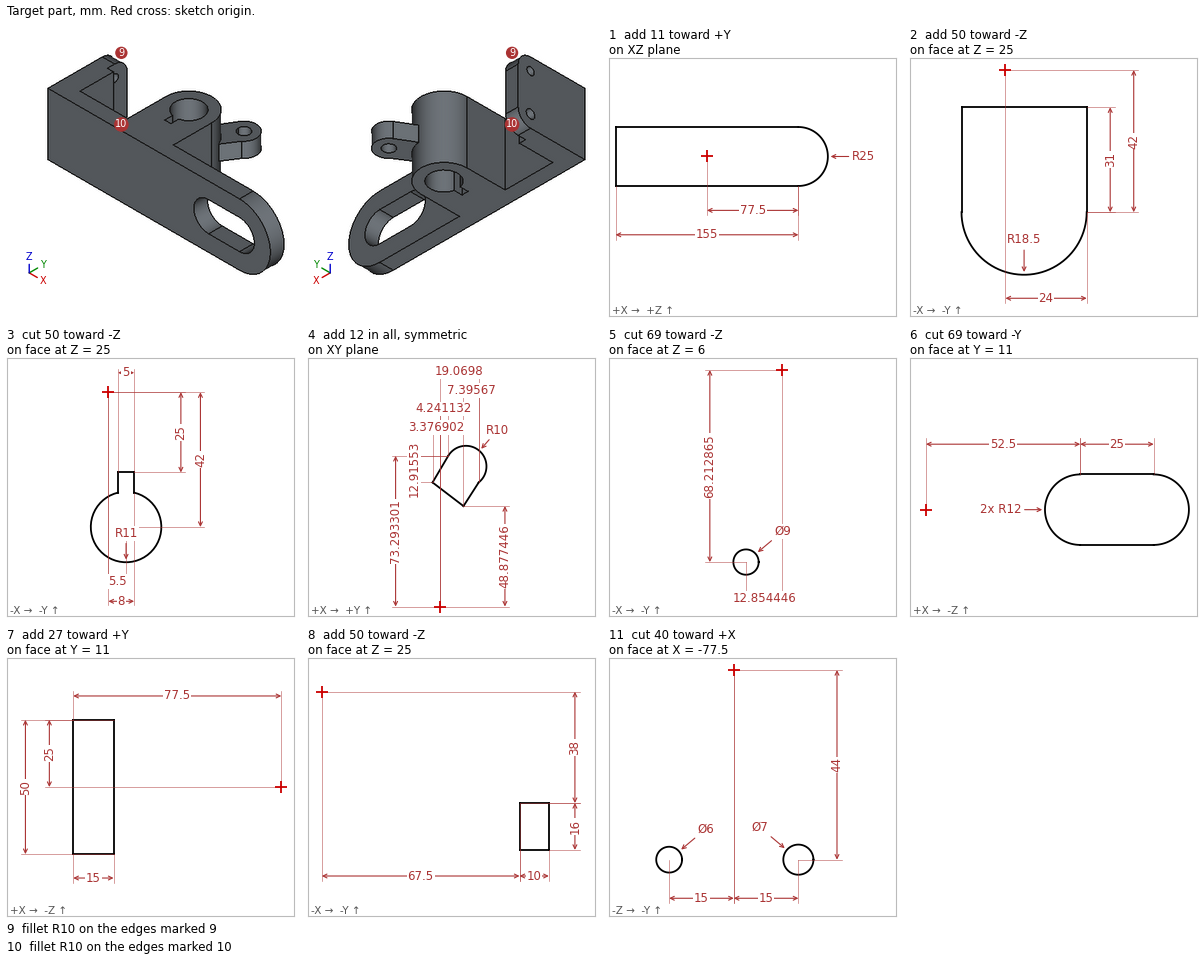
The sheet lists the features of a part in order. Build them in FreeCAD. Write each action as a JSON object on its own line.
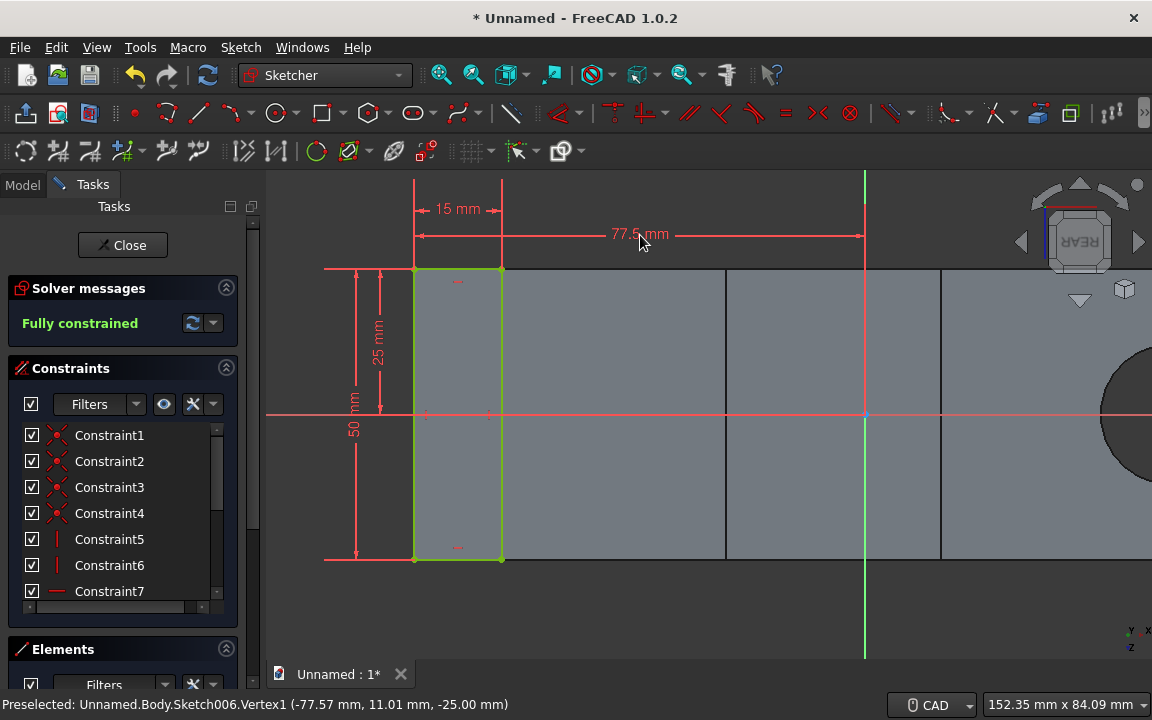
{"action": "left_click", "coordinate": [123, 245]}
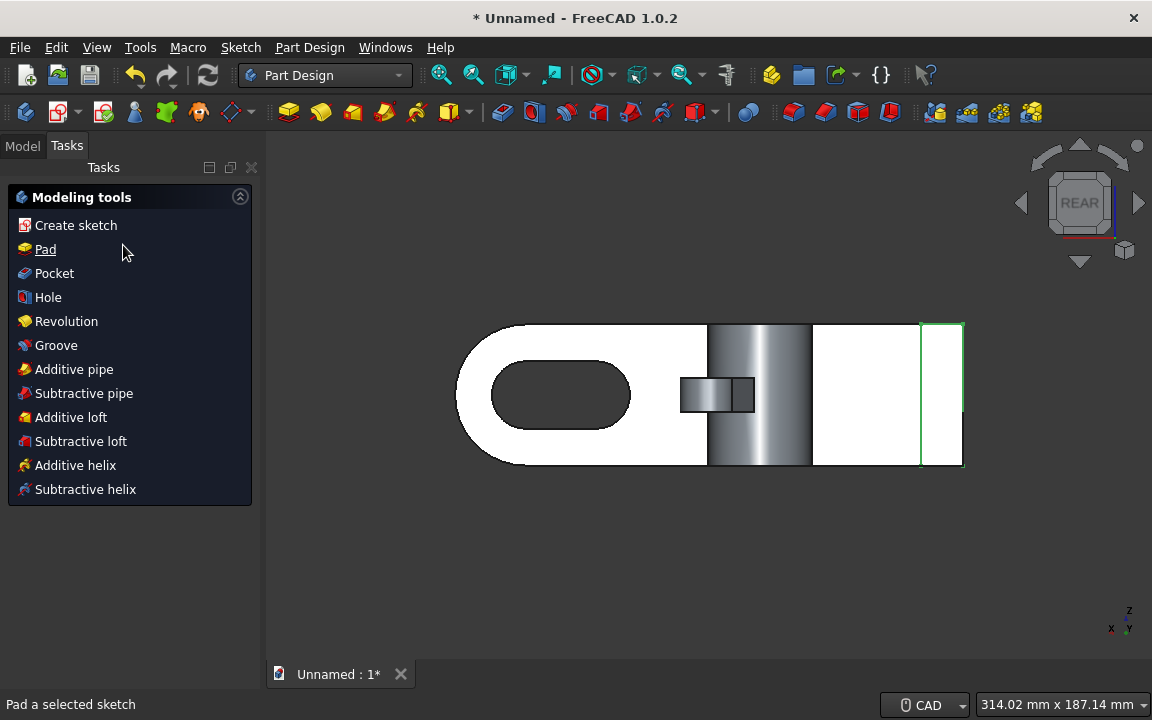
{"action": "left_click", "coordinate": [290, 112]}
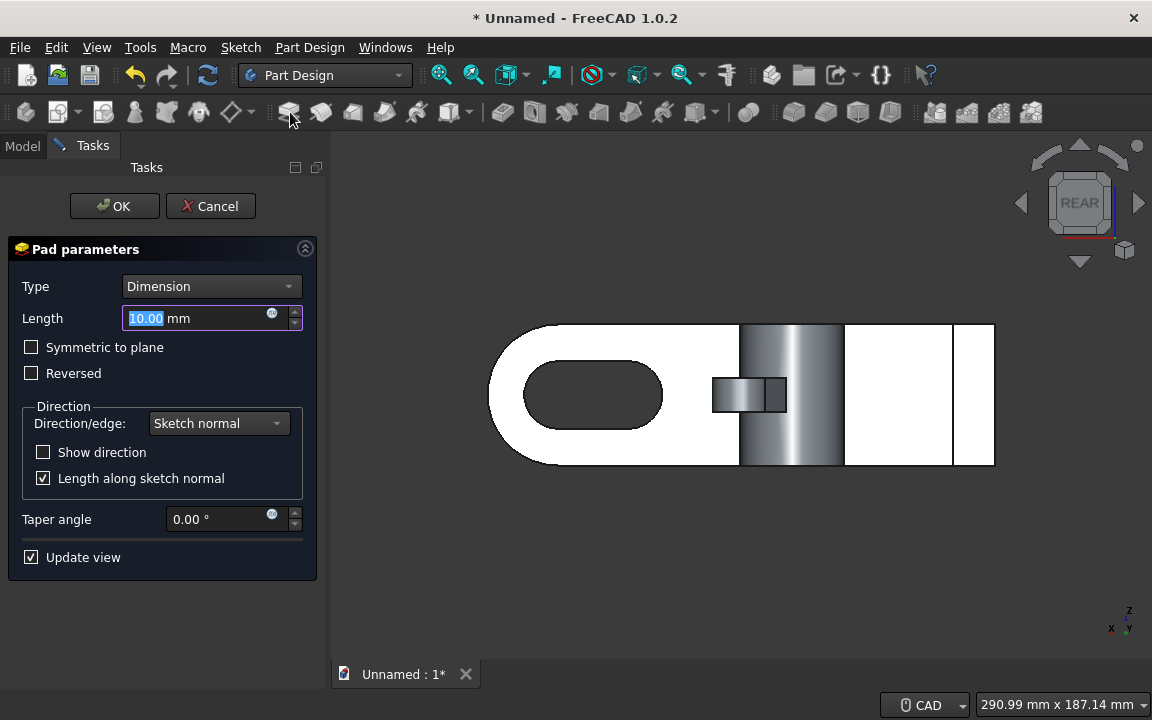
{"action": "type", "text": "27"}
{"action": "key", "text": "Tab"}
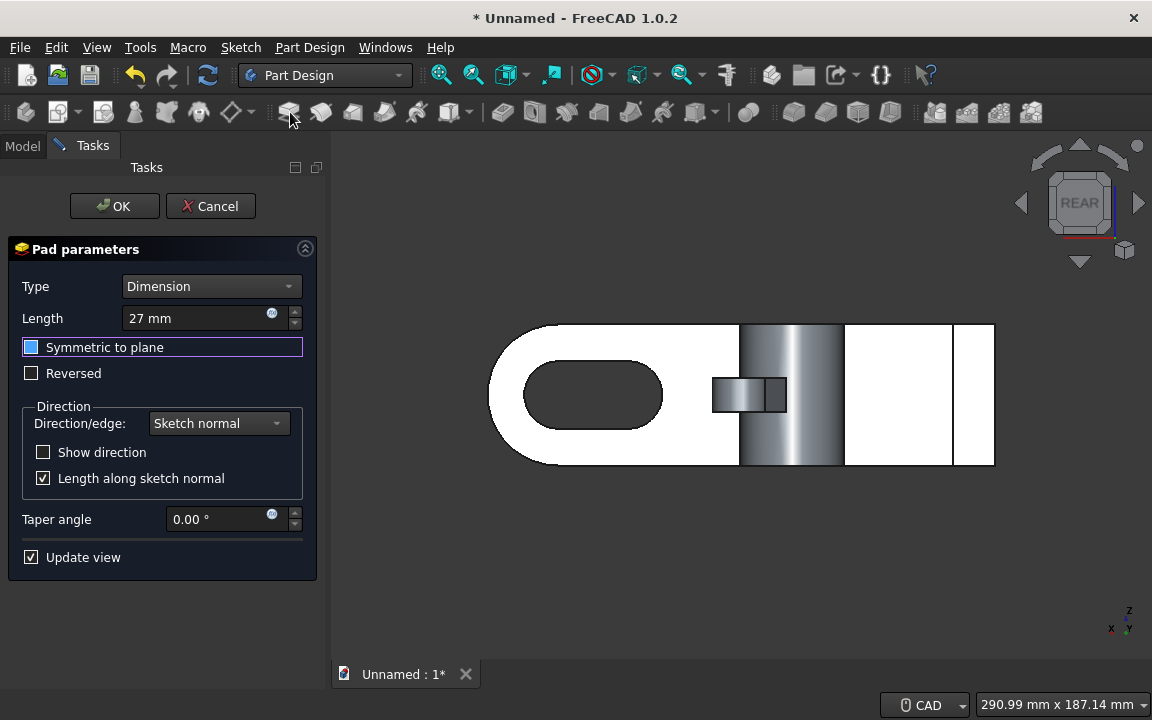
{"action": "left_click", "coordinate": [115, 206]}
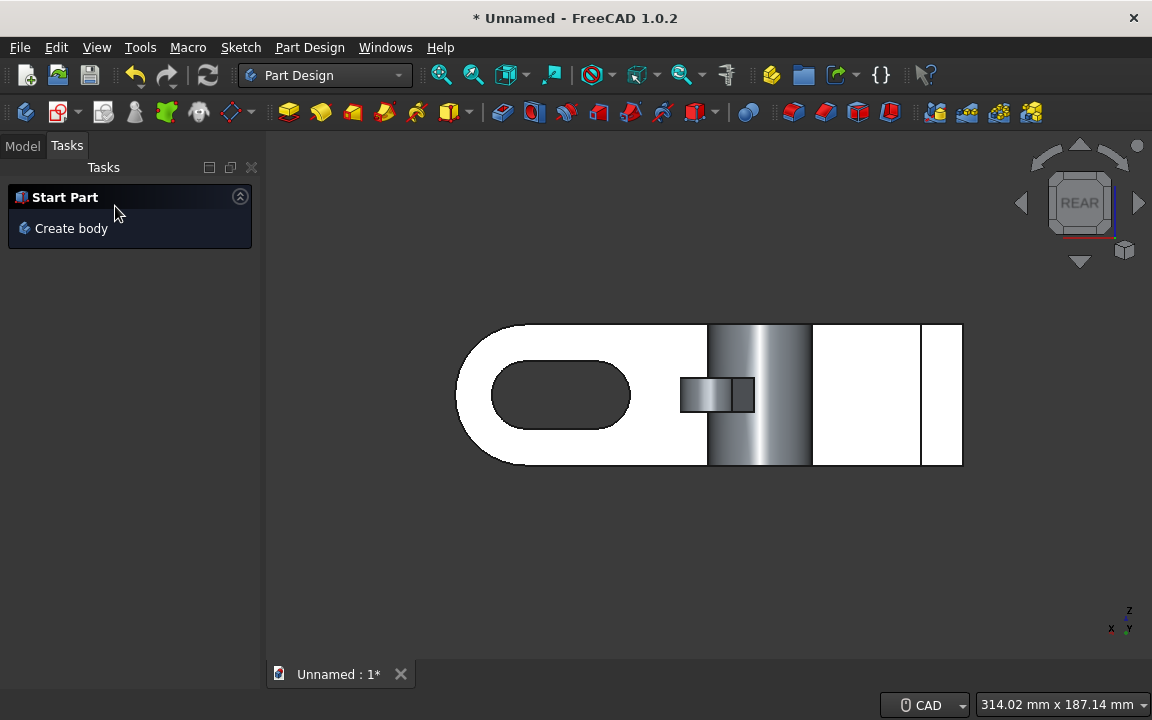
{"action": "key", "text": "0"}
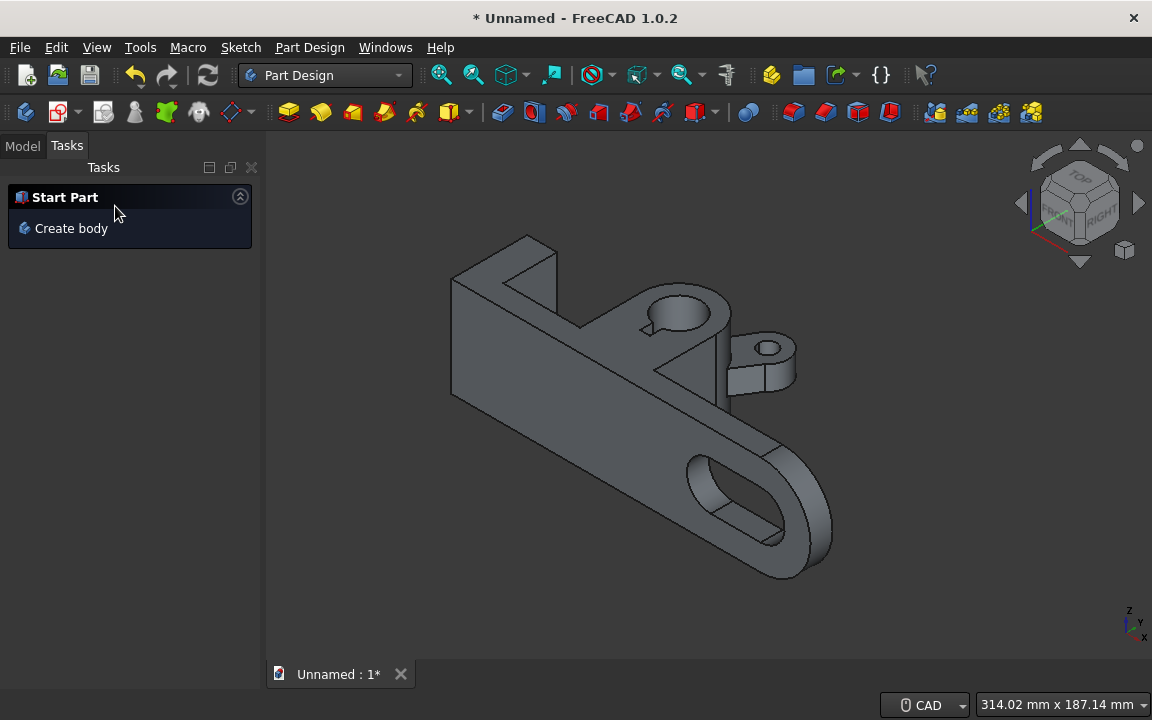
{"action": "left_click", "coordinate": [632, 352]}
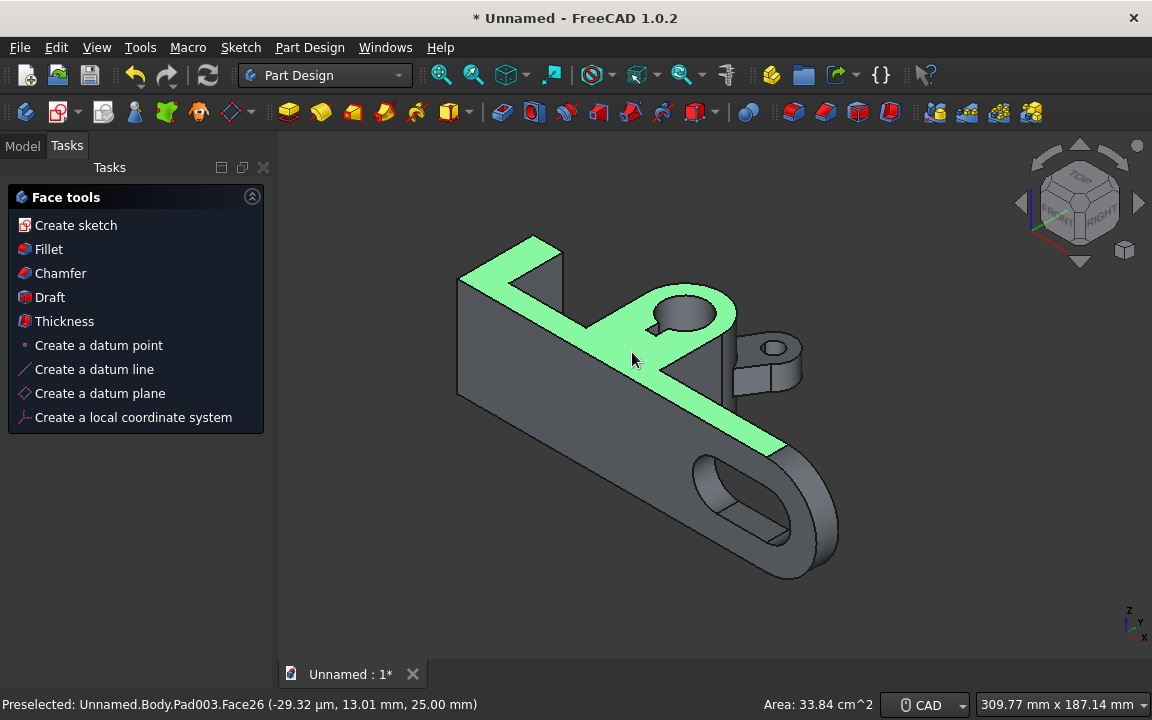
{"action": "left_click", "coordinate": [58, 112]}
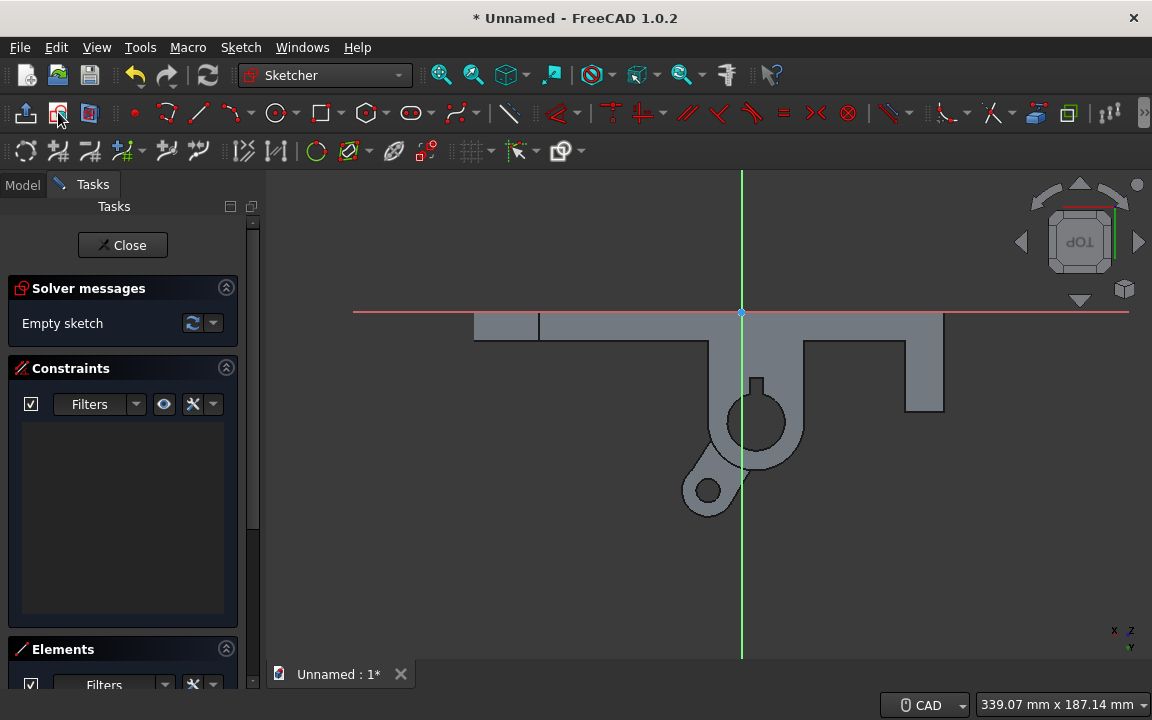
{"action": "scroll", "coordinate": [977, 435], "scroll_direction": "up", "scroll_amount": 10}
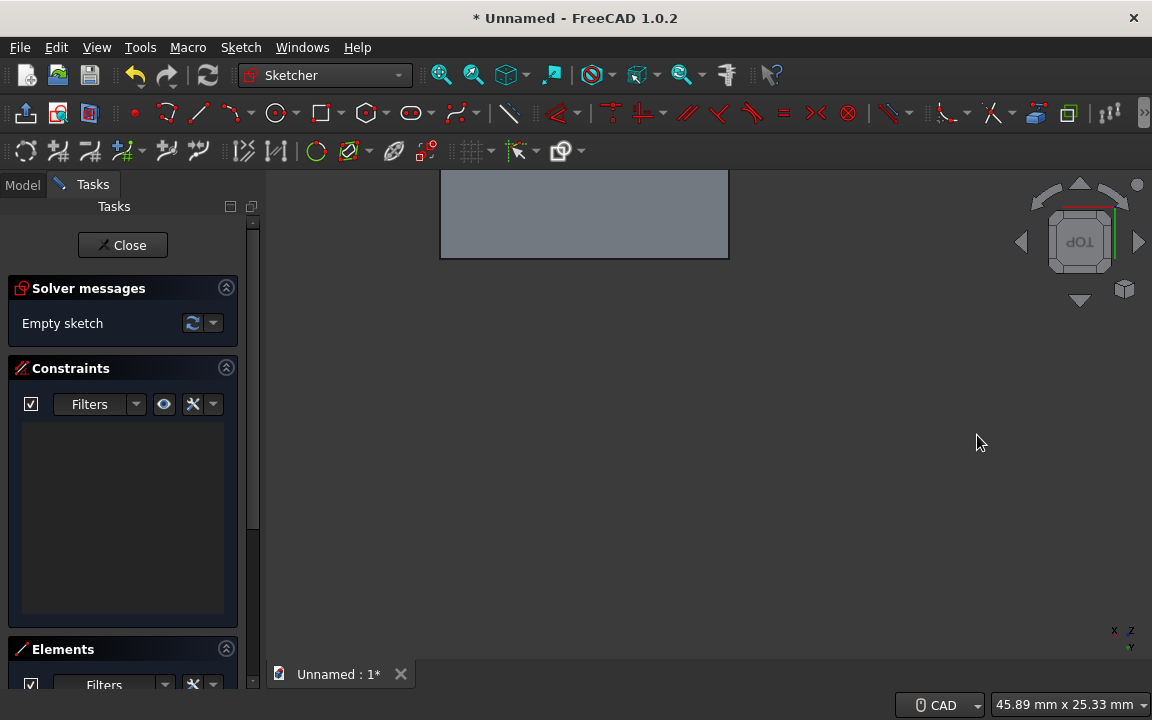
{"action": "left_click", "coordinate": [322, 114]}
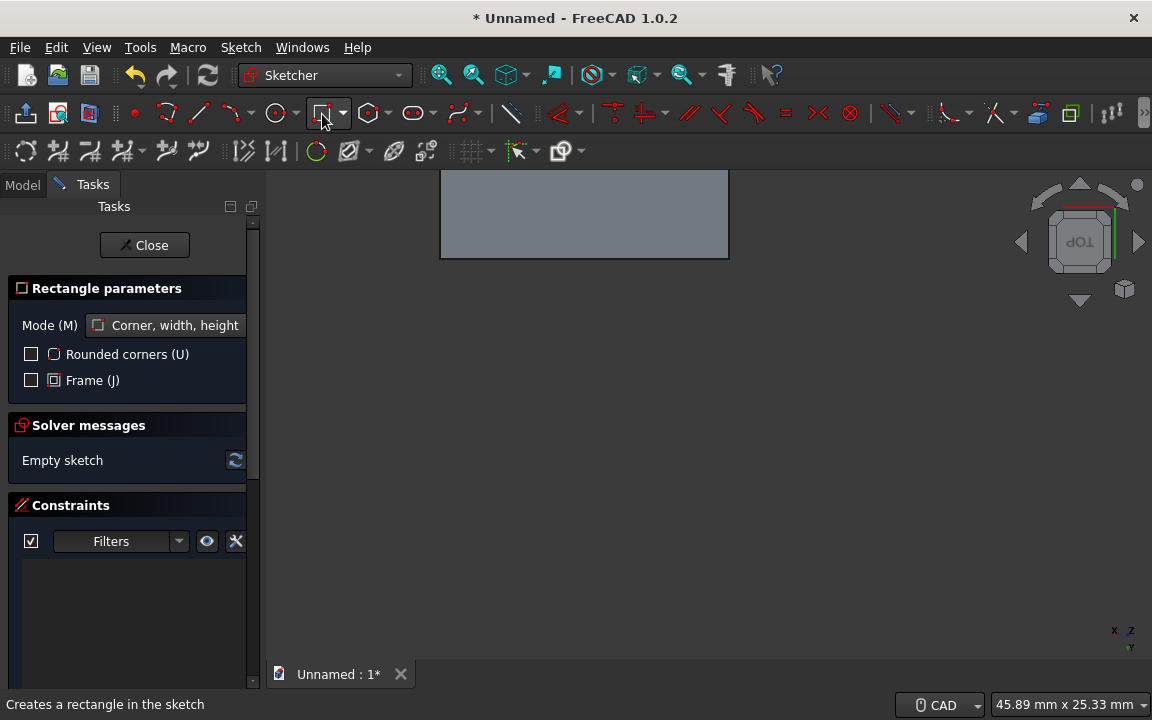
{"action": "left_click", "coordinate": [536, 259]}
{"action": "mouse_move", "coordinate": [729, 568]}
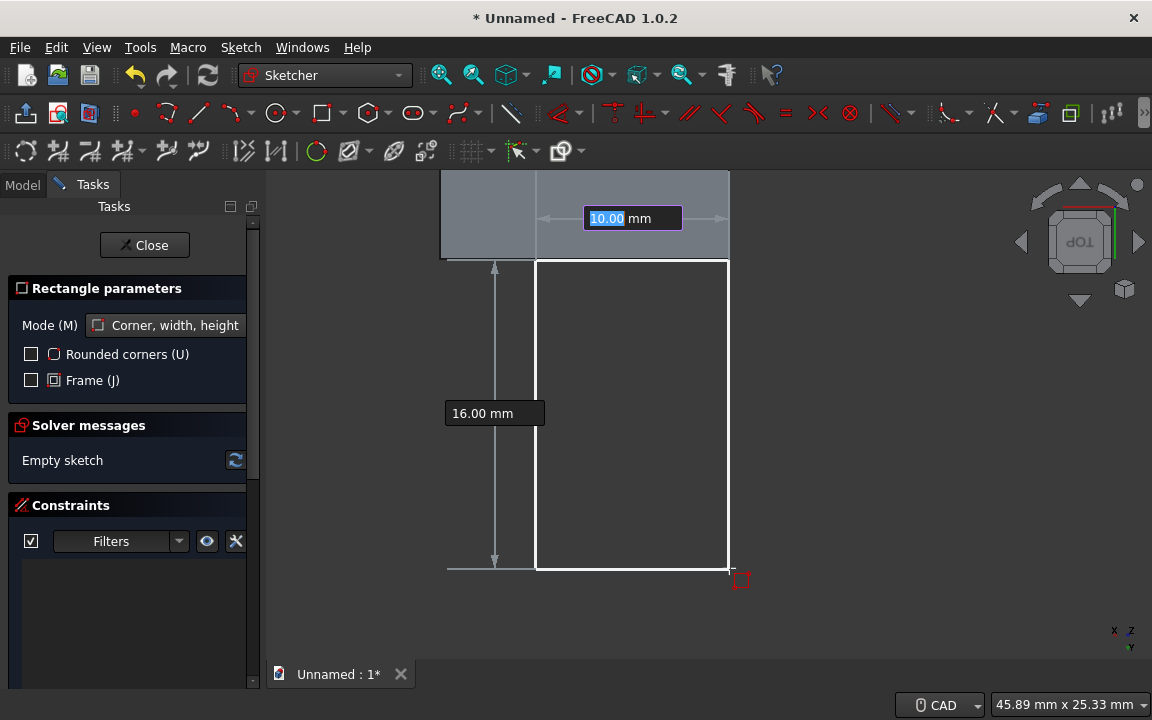
{"action": "type", "text": "10"}
{"action": "key", "text": "Tab"}
{"action": "type", "text": "16"}
{"action": "key", "text": "Return"}
{"action": "key", "text": "Escape"}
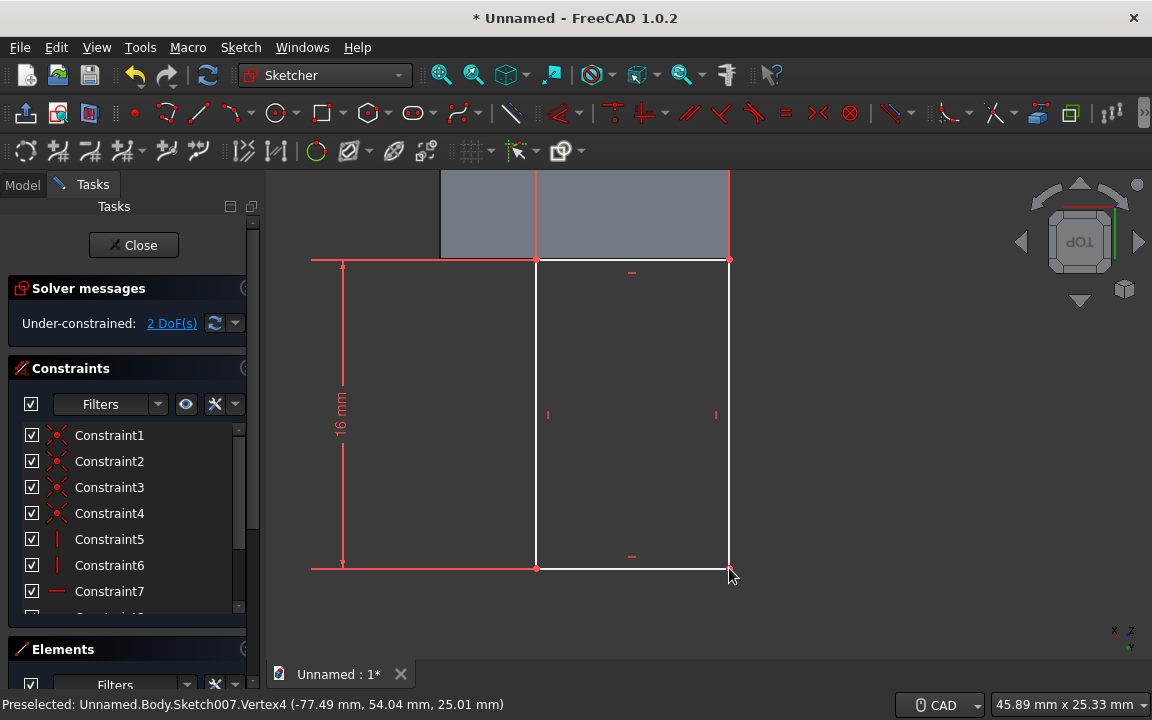
{"action": "left_click", "coordinate": [558, 114]}